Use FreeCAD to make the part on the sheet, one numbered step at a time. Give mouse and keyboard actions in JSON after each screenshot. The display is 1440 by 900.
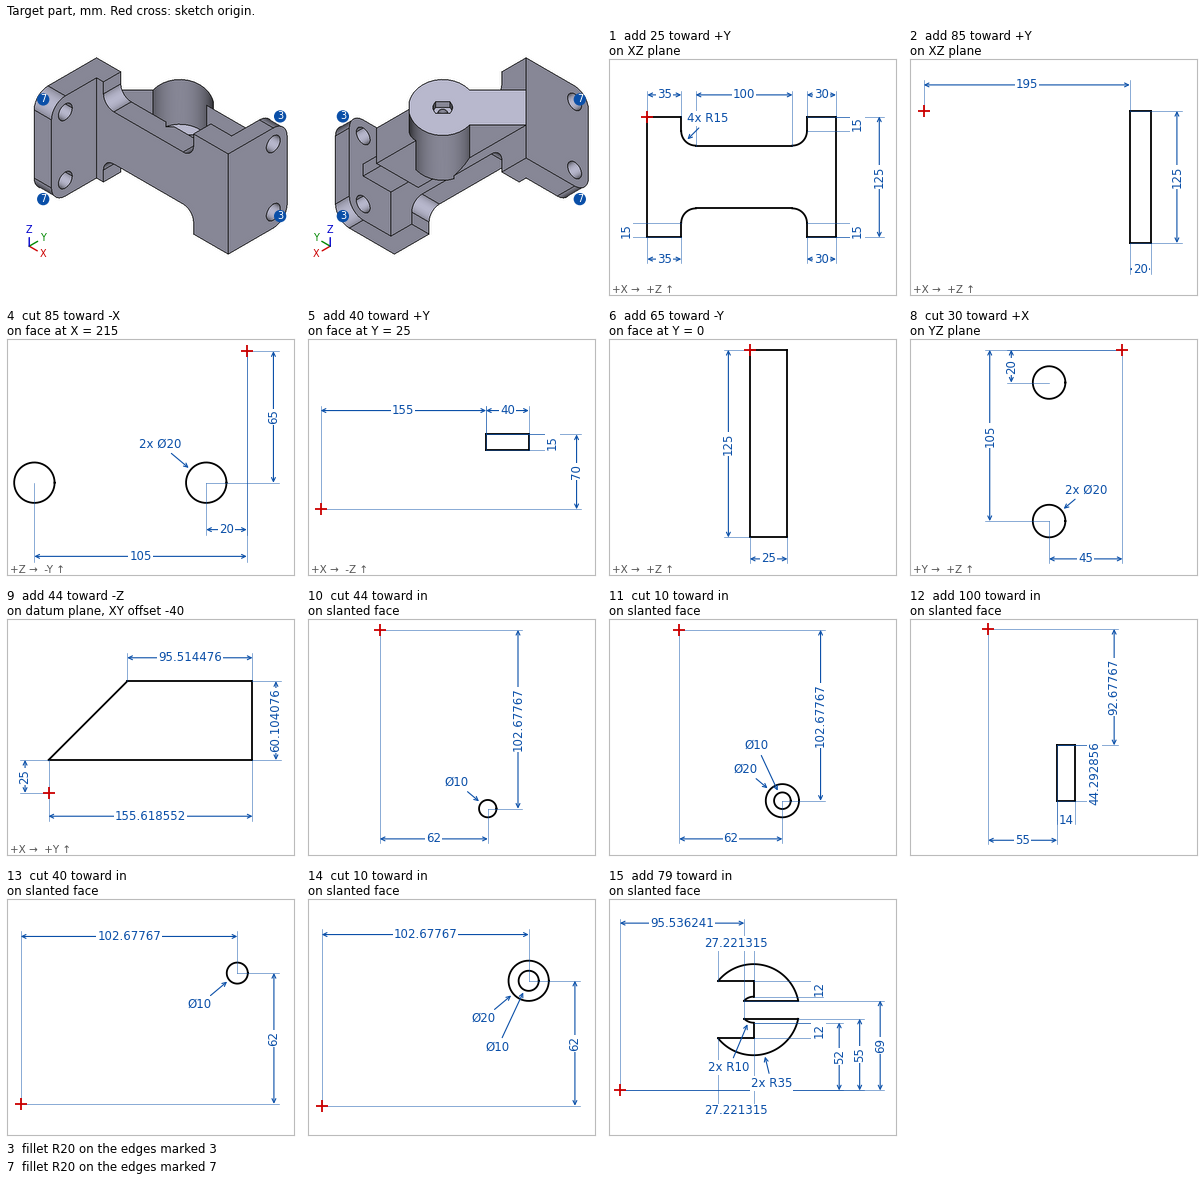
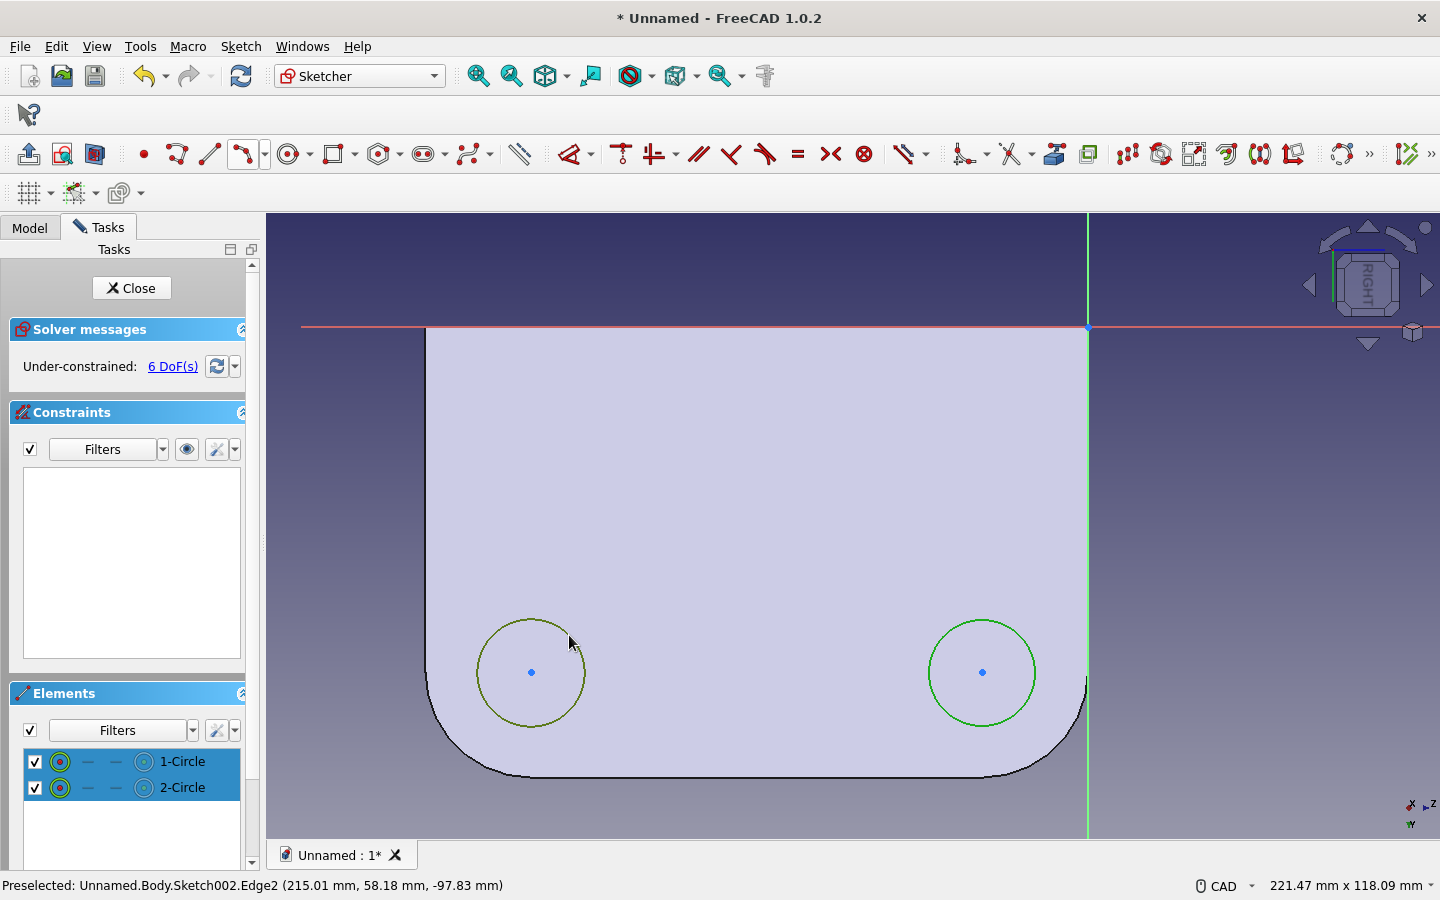
{"action": "left_click", "coordinate": [798, 154]}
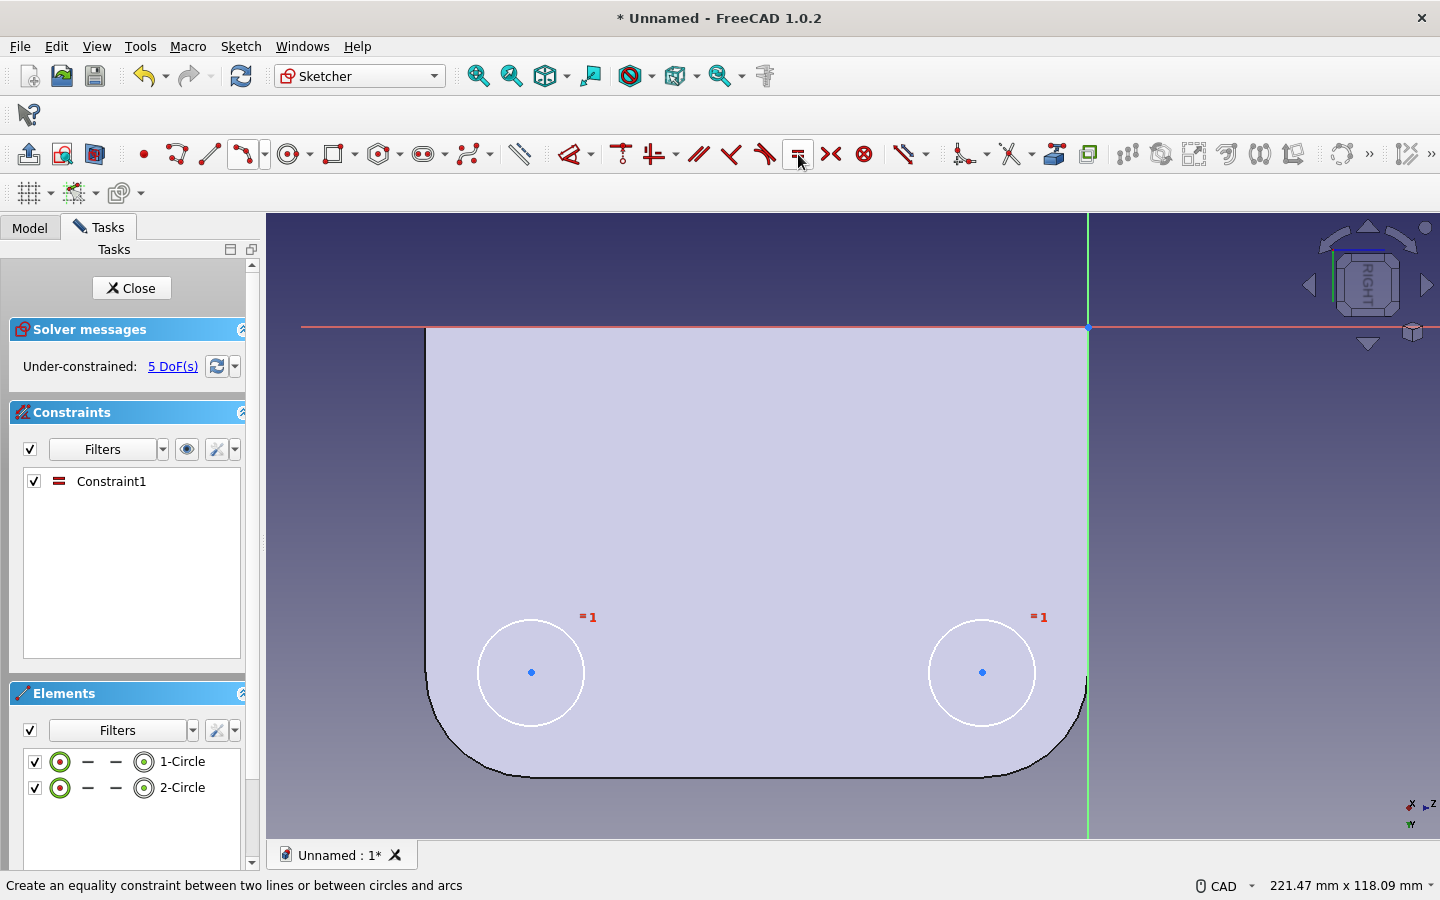
{"action": "left_click", "coordinate": [982, 673]}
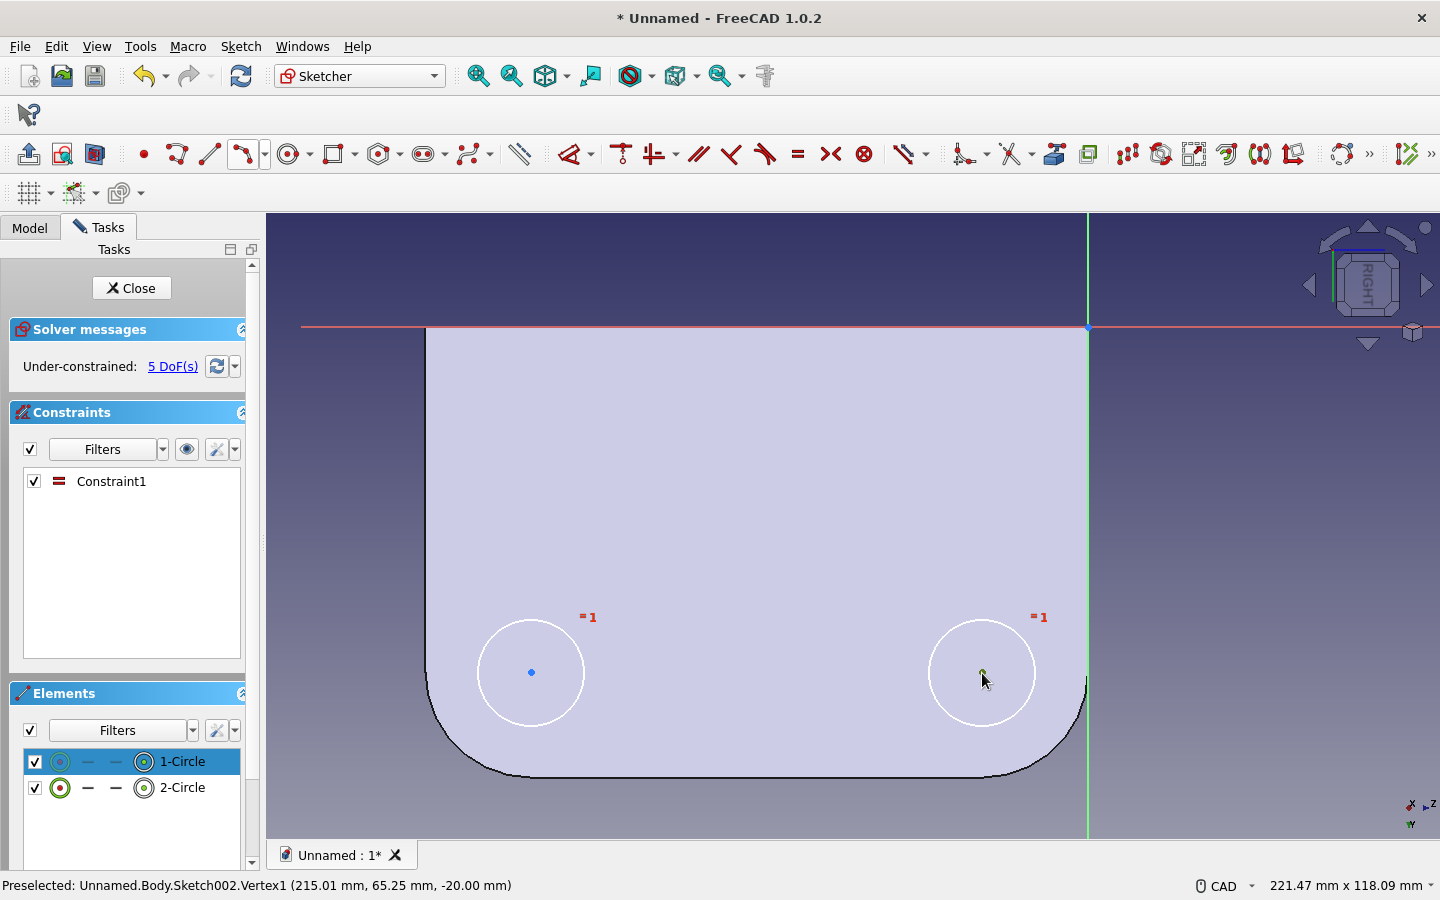
{"action": "left_click", "coordinate": [531, 673]}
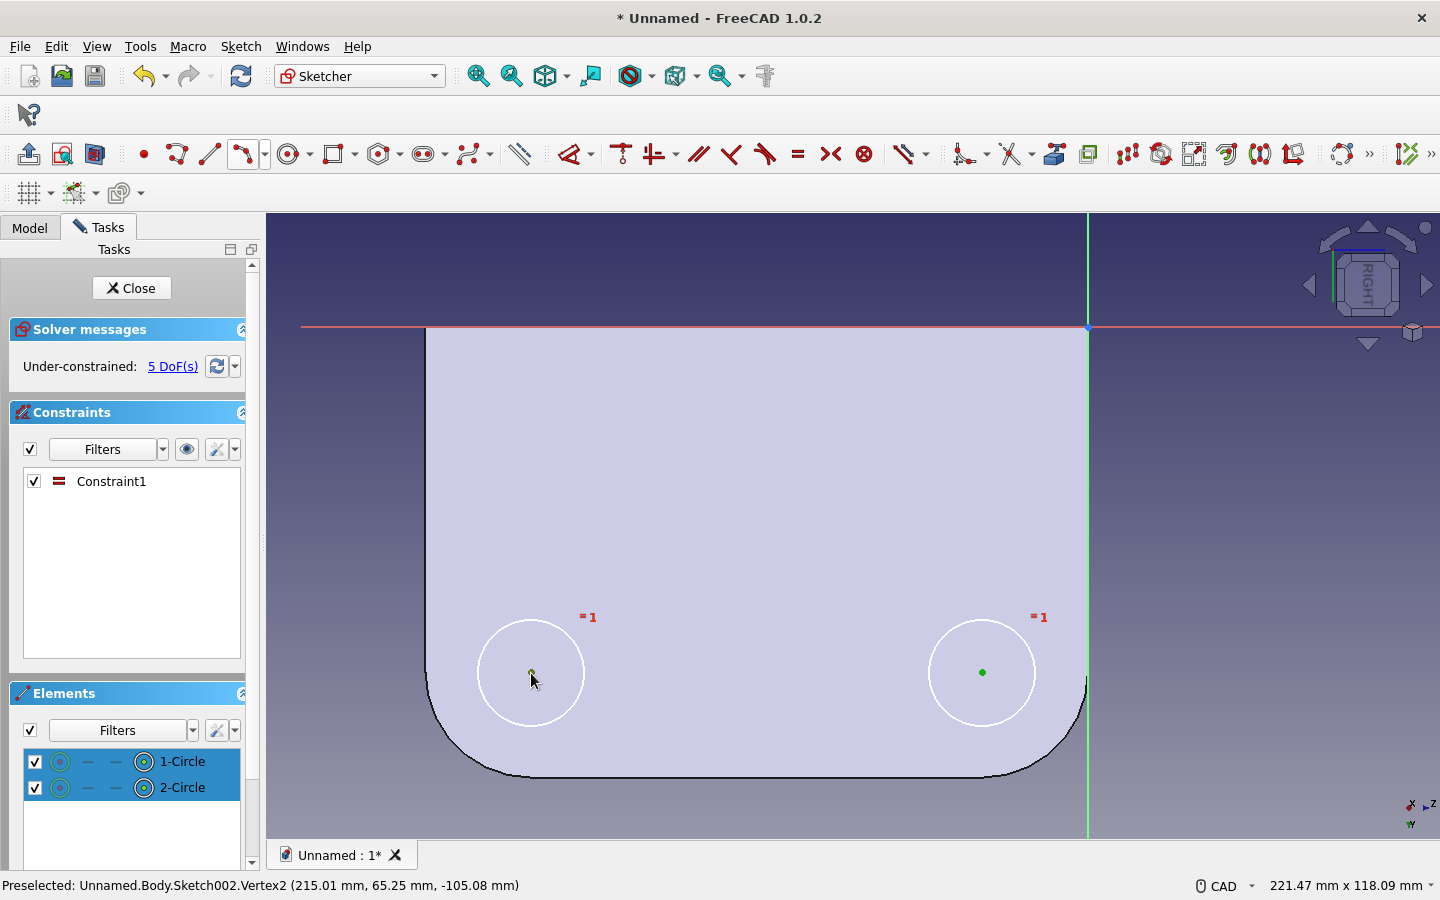
{"action": "key", "text": "h"}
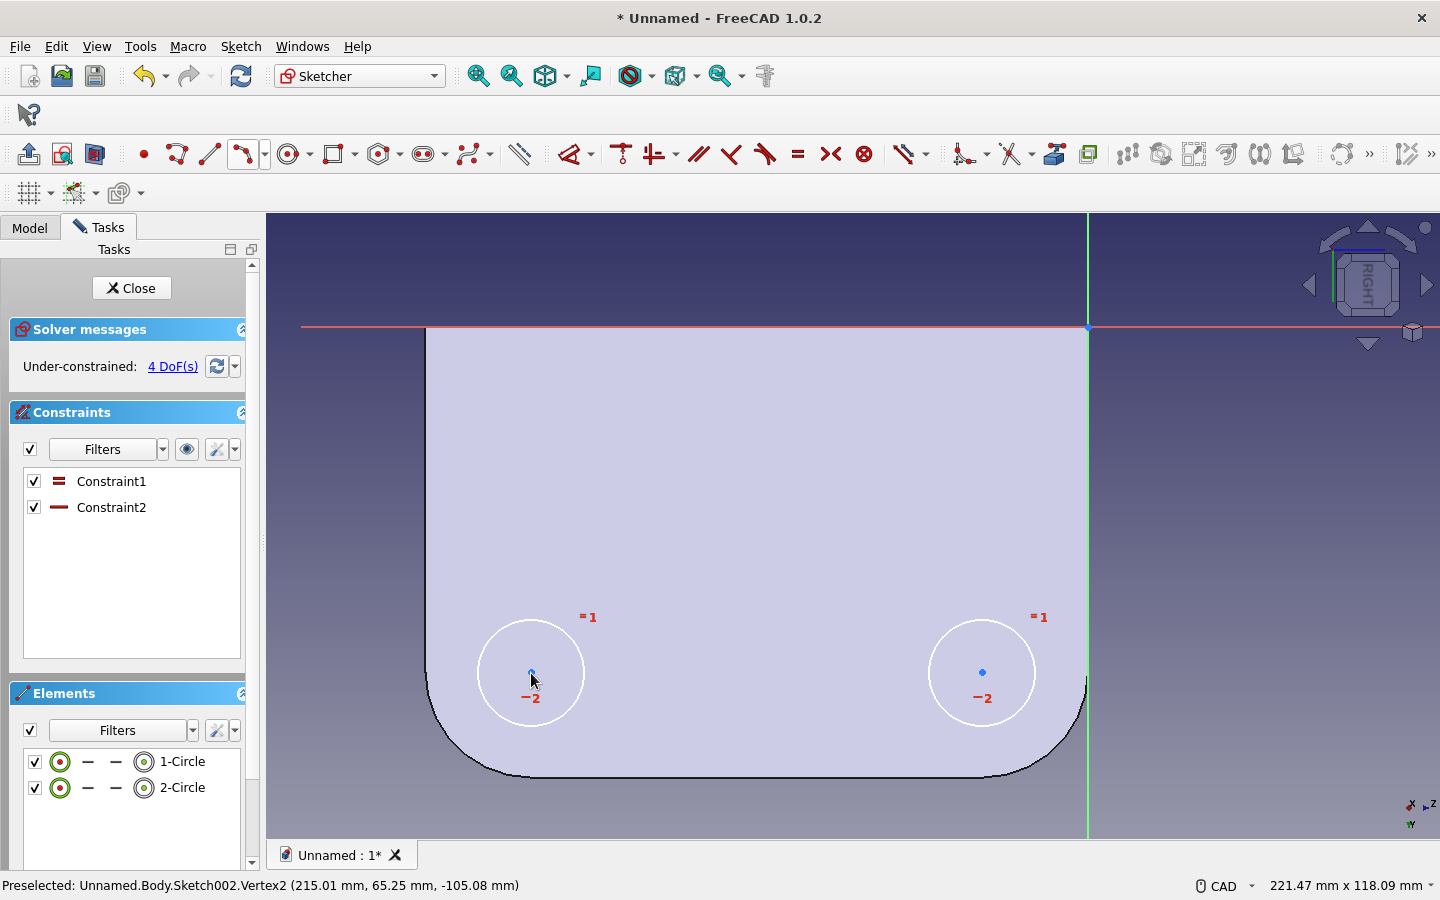
{"action": "key", "text": "d"}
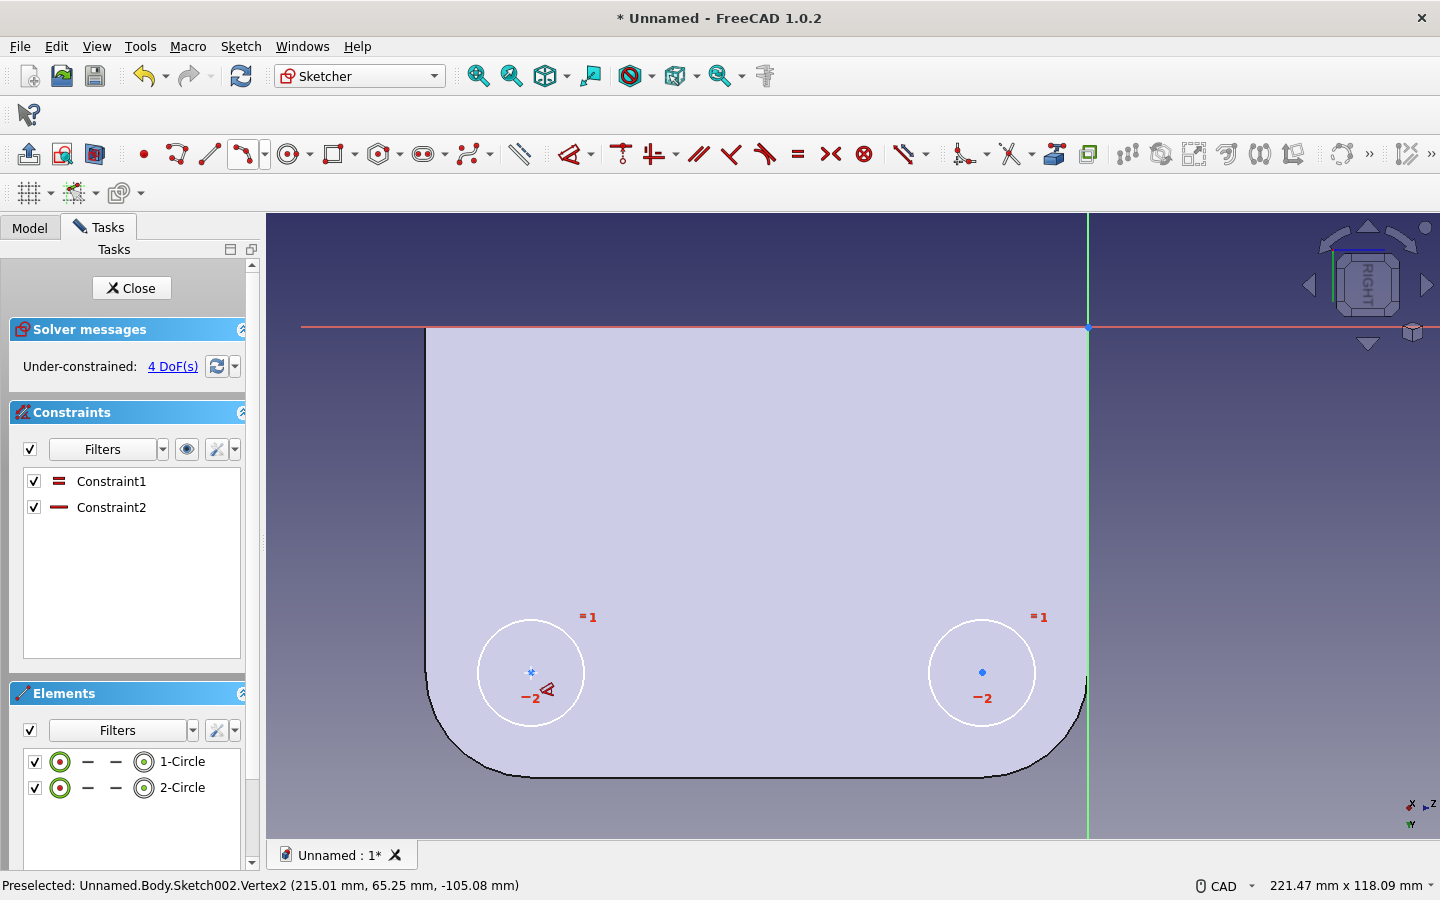
{"action": "left_click", "coordinate": [1019, 635]}
{"action": "left_click", "coordinate": [1041, 612]}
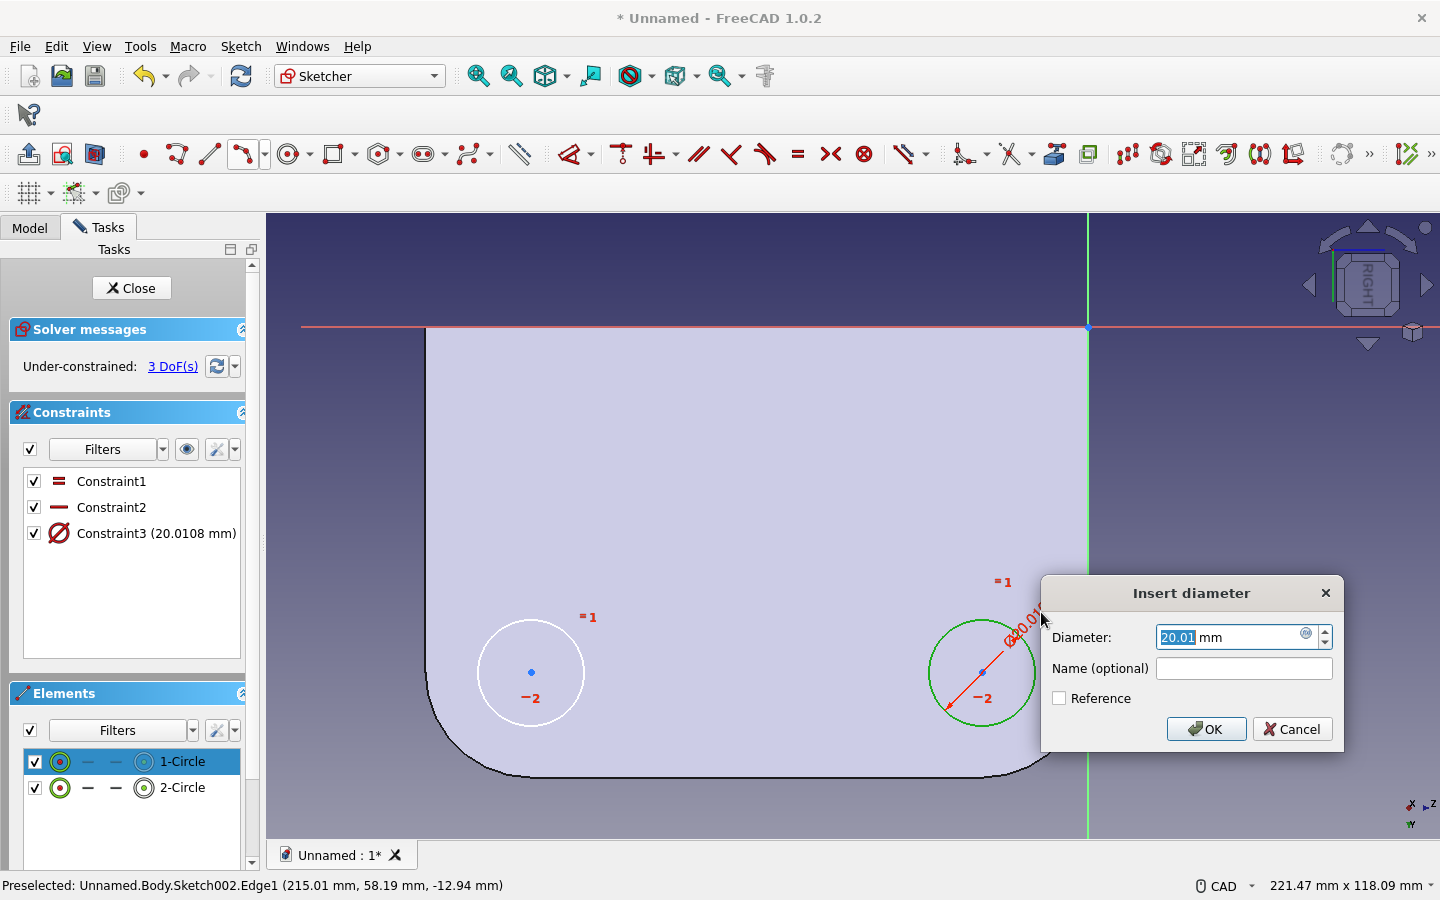
{"action": "type", "text": "20"}
{"action": "key", "text": "Return"}